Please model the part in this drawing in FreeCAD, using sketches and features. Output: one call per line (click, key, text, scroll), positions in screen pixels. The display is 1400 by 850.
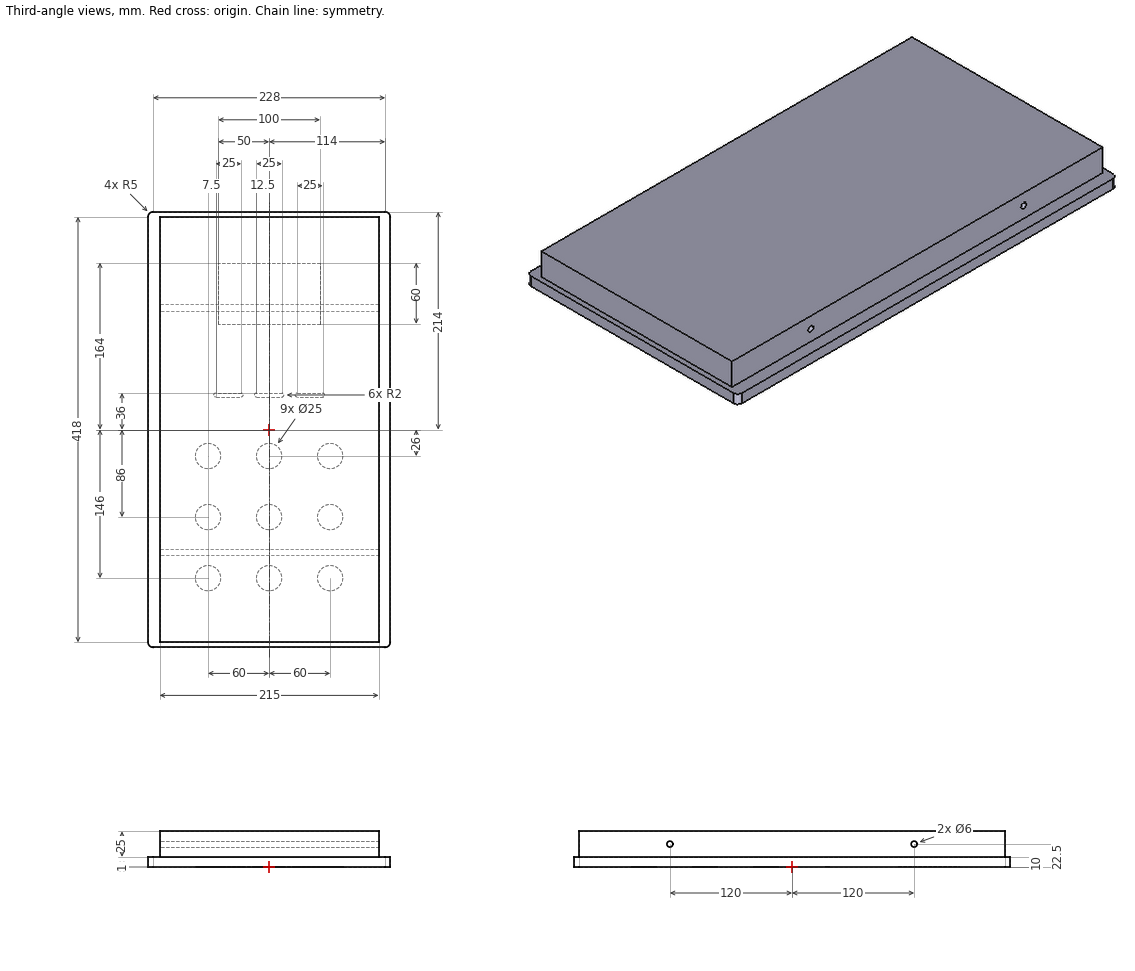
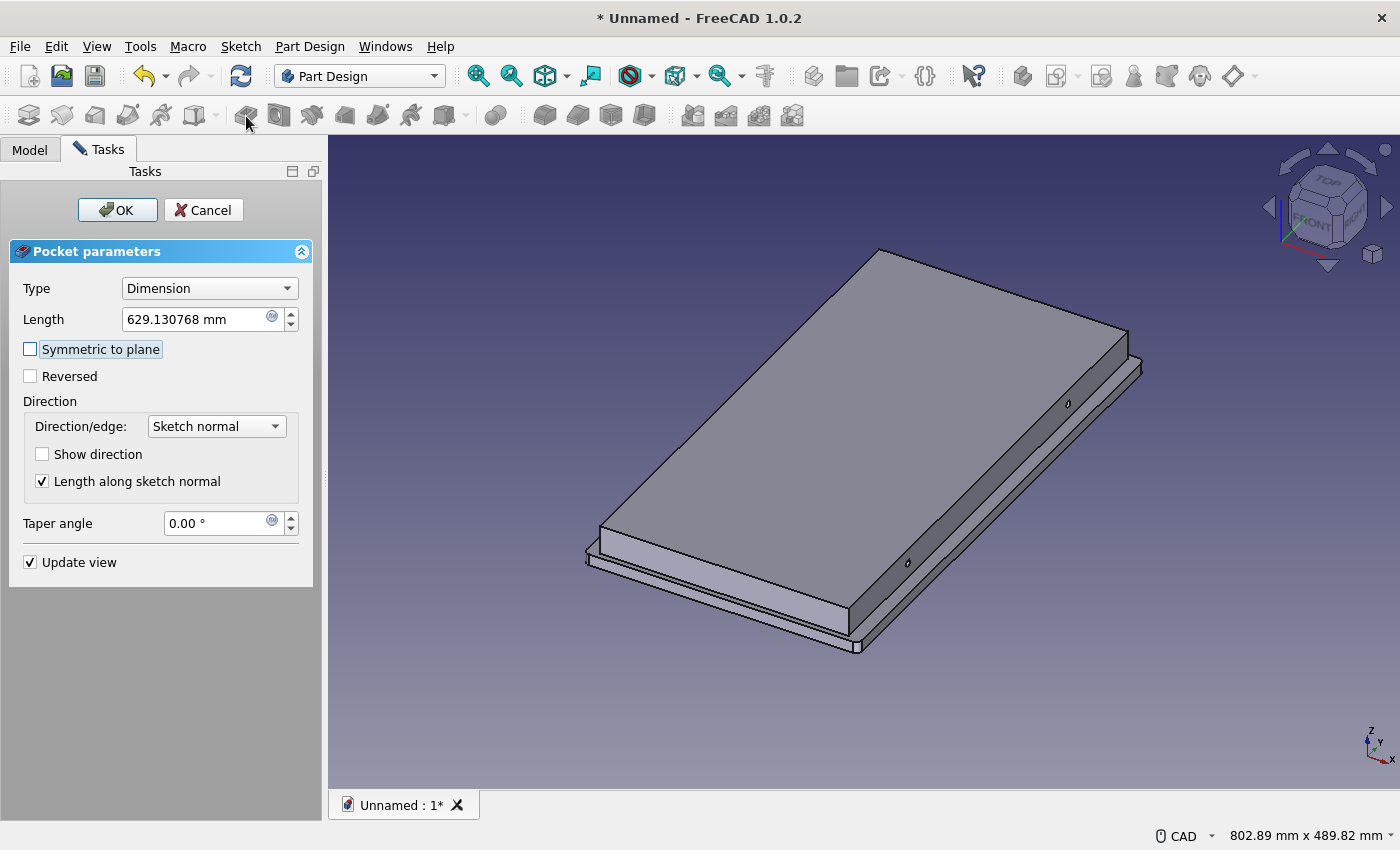
click(31, 349)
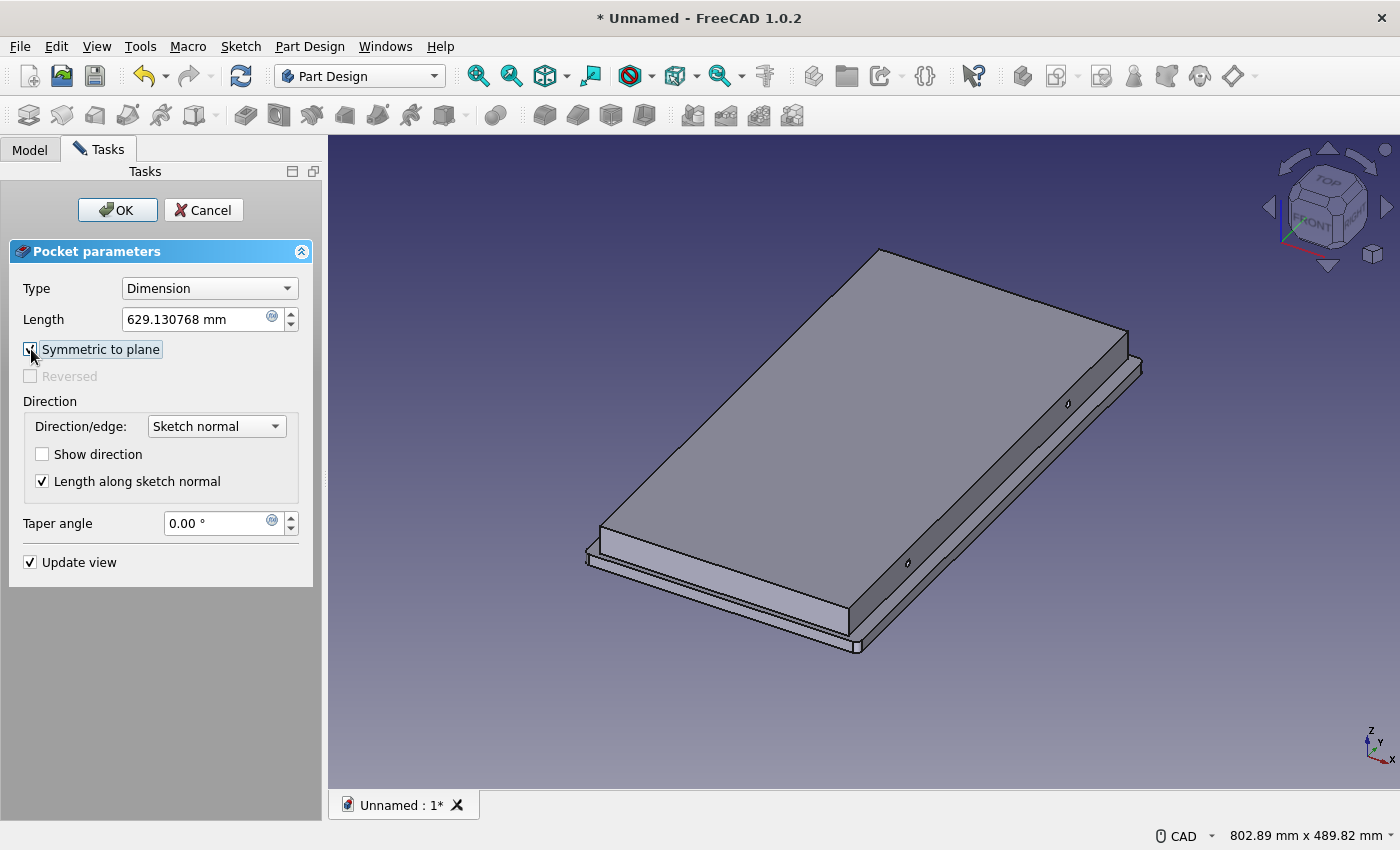
click(118, 210)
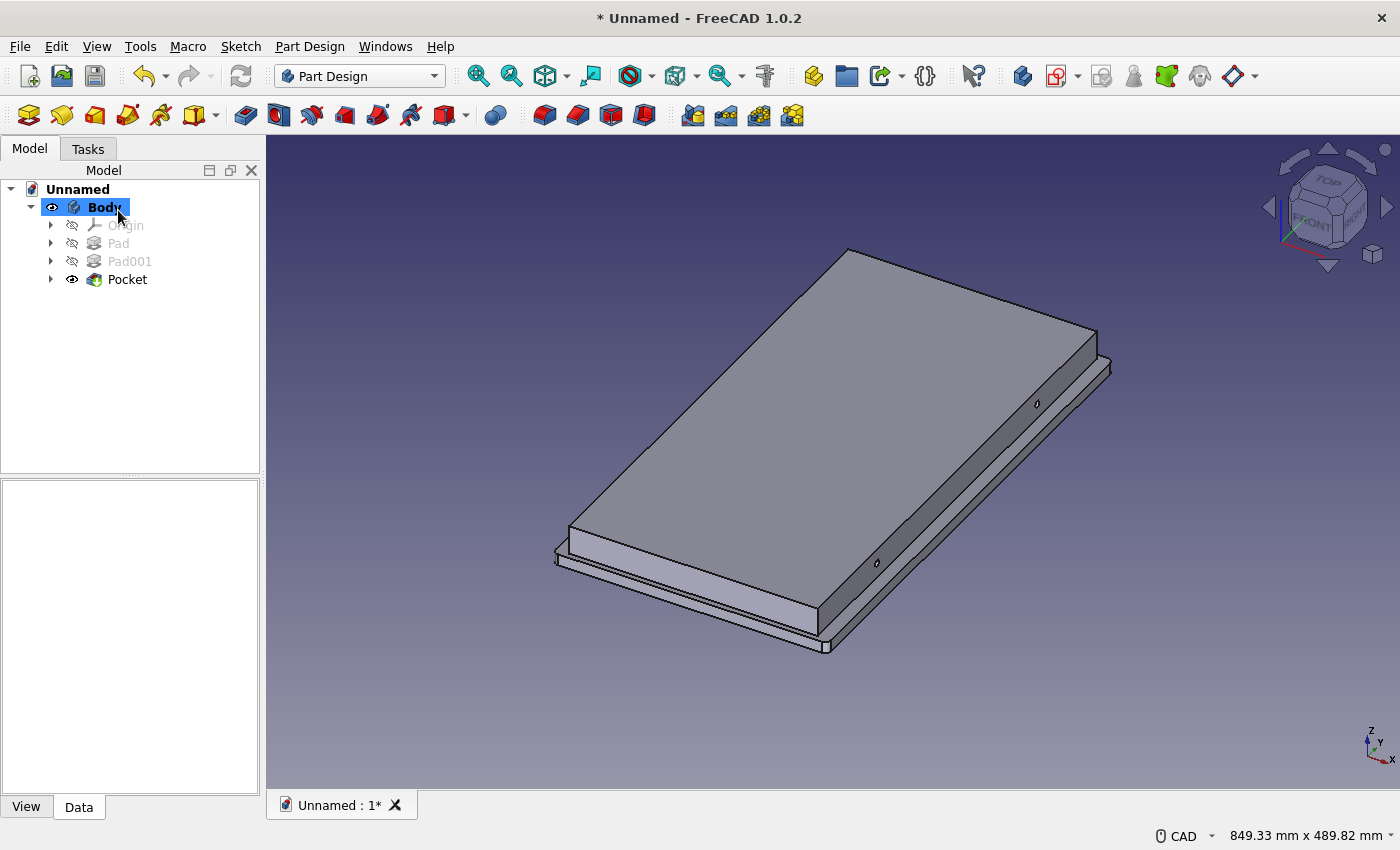
click(1056, 76)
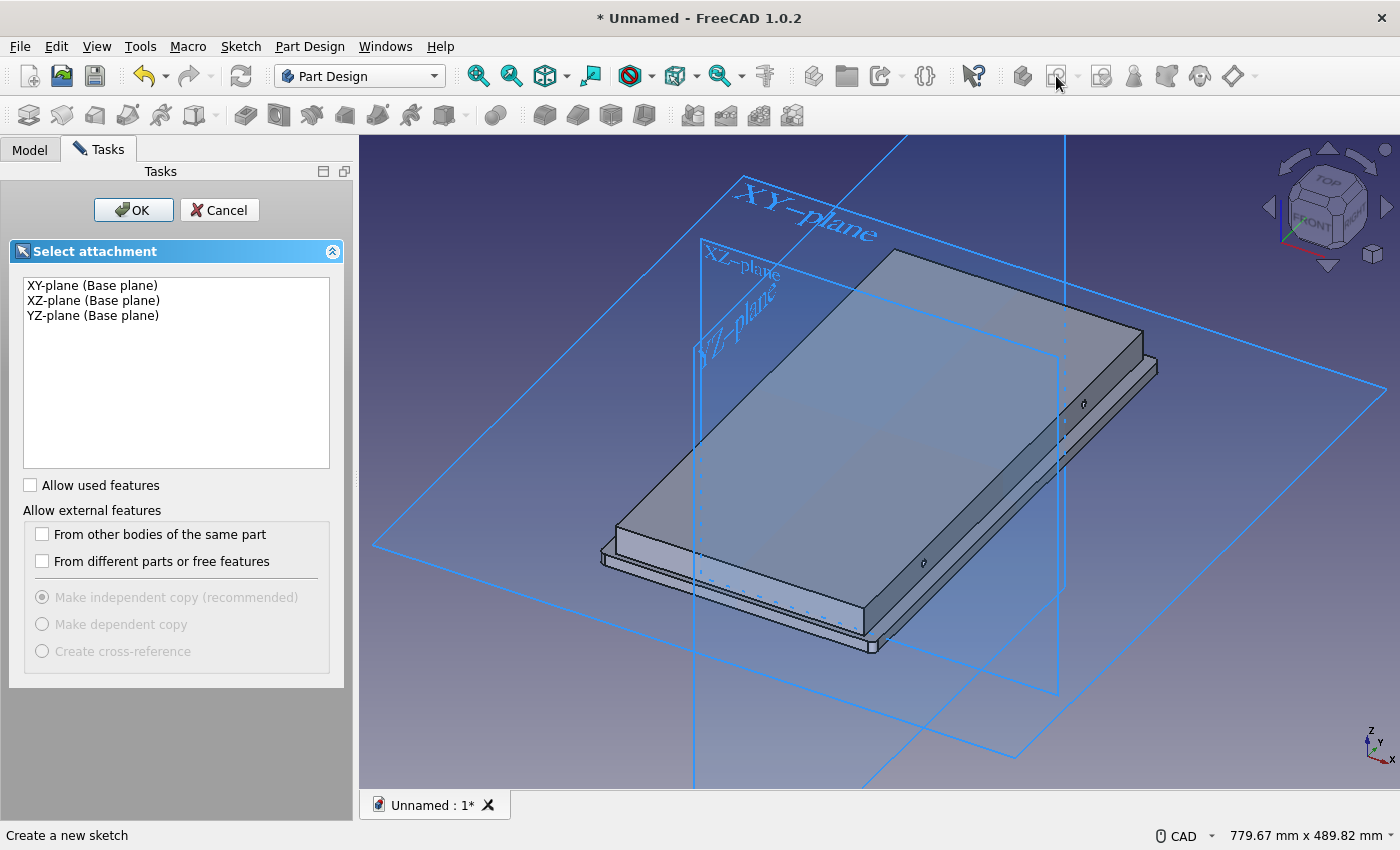
click(84, 286)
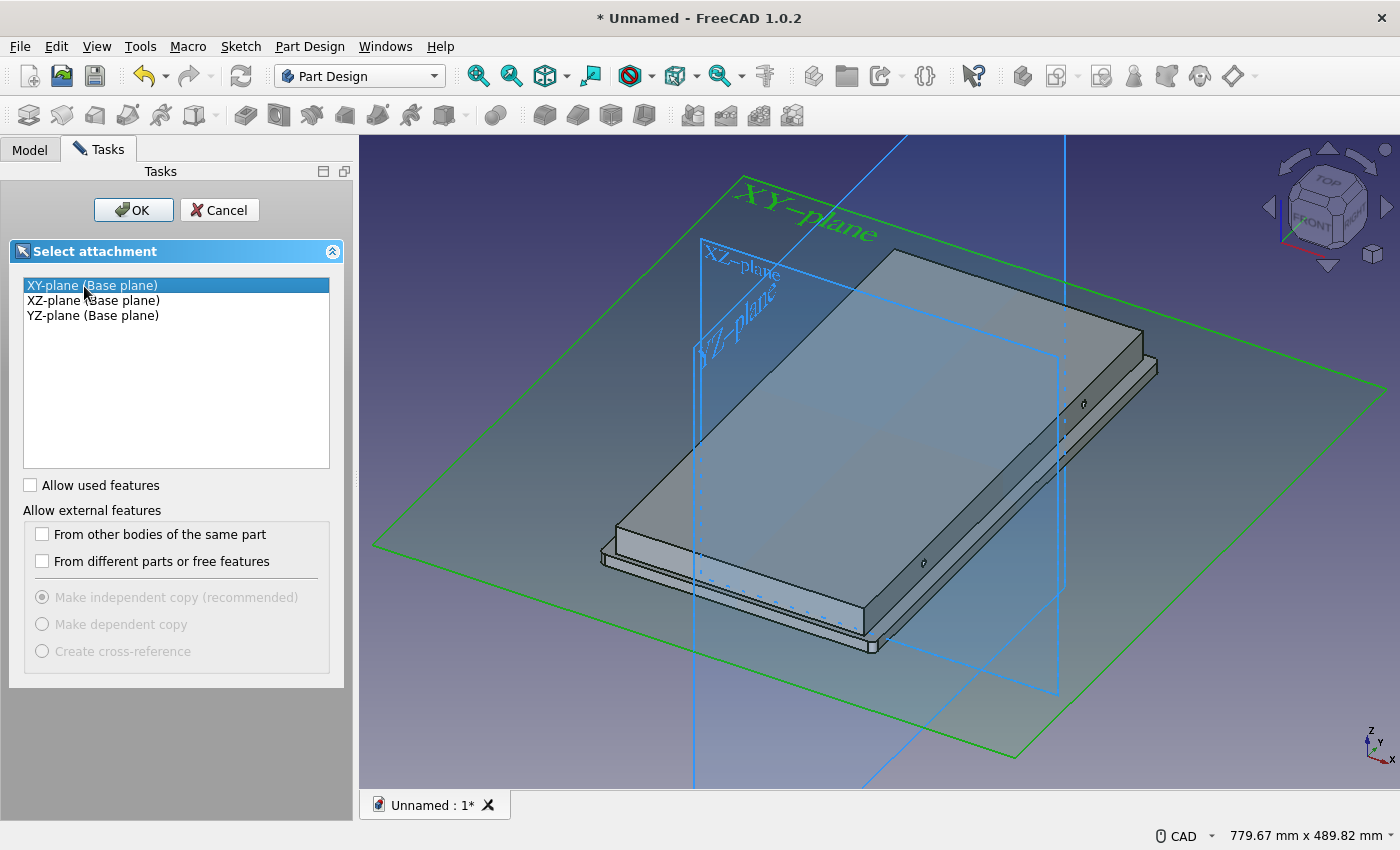
click(134, 210)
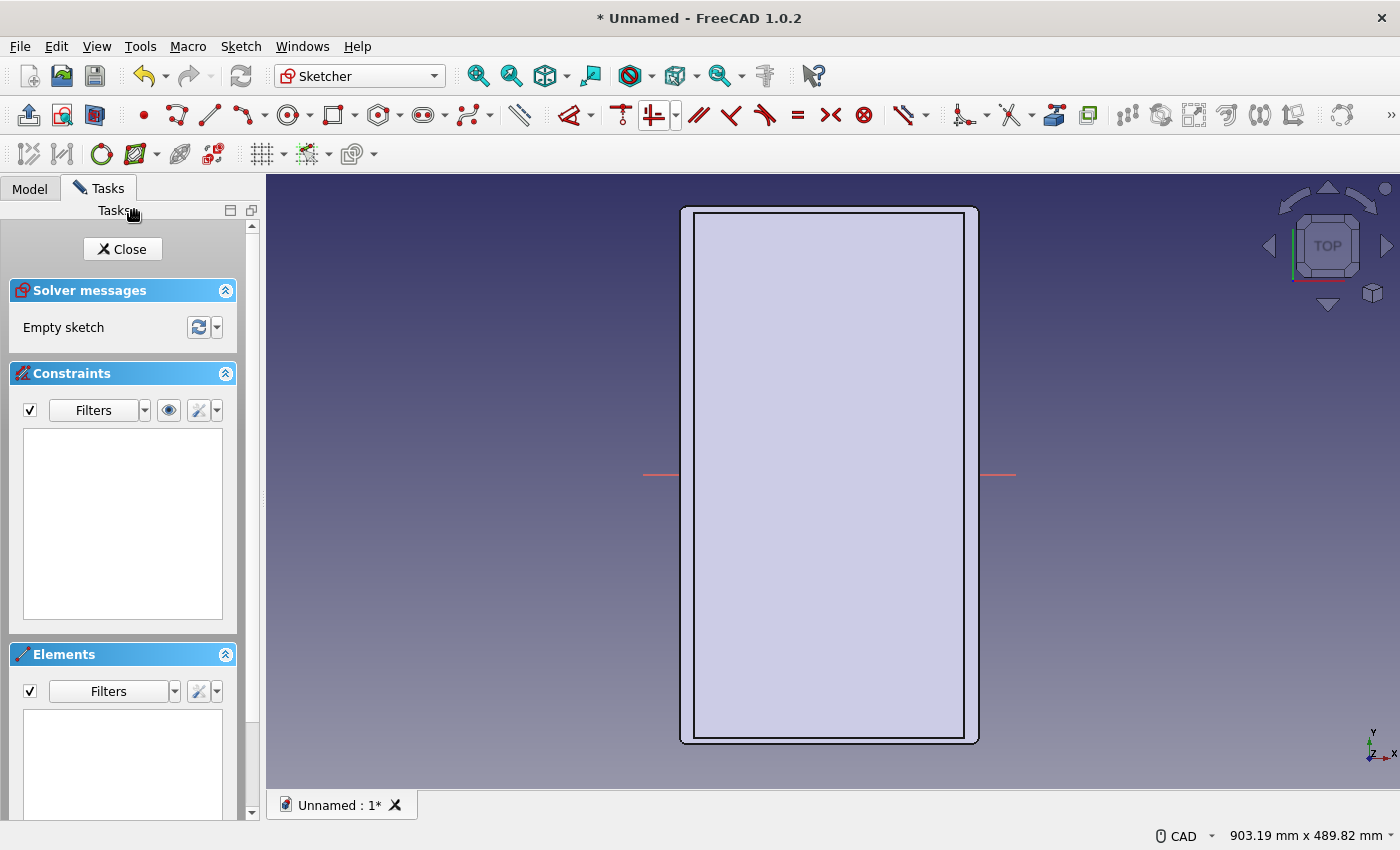
key(q)
key(s)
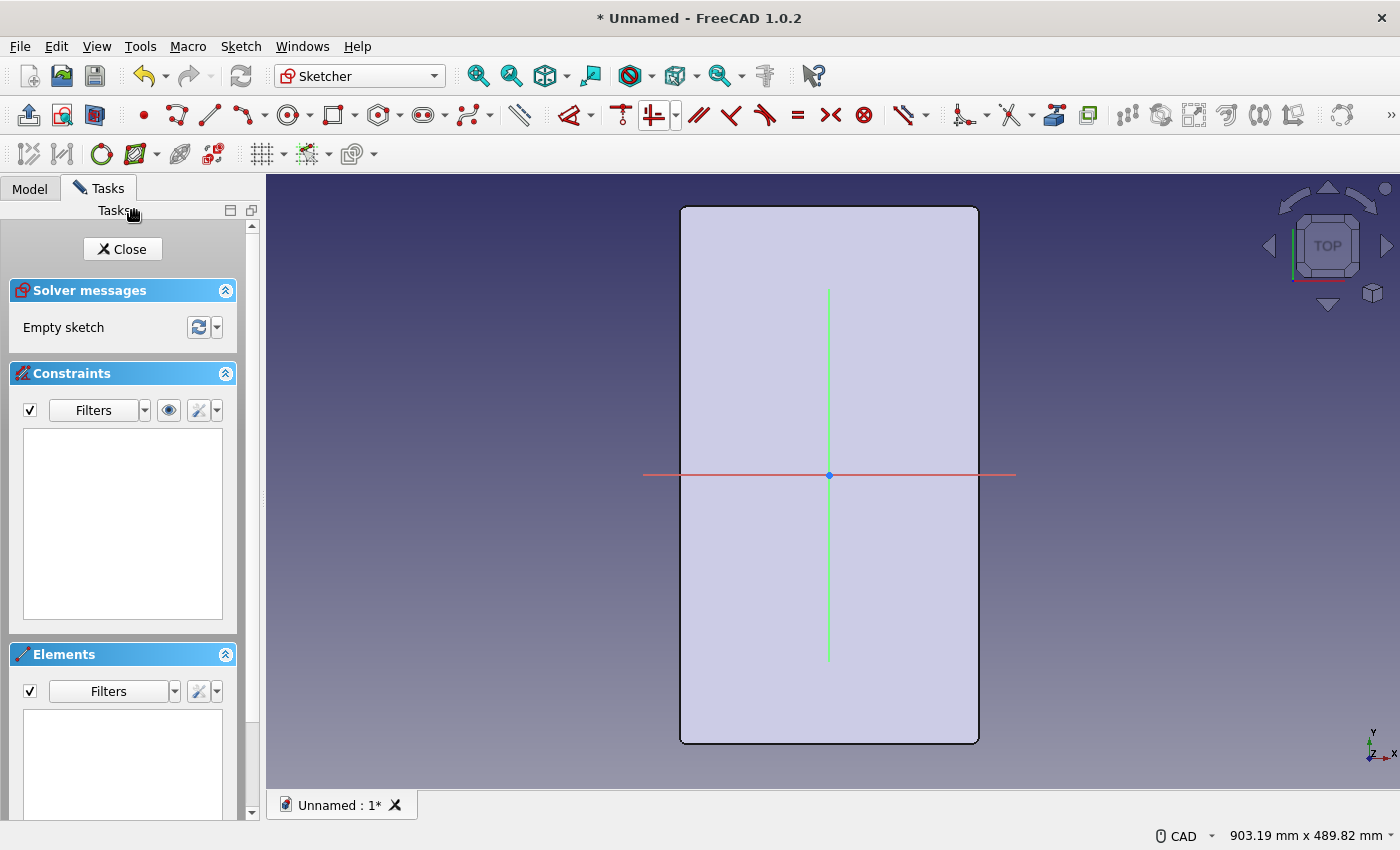
click(332, 116)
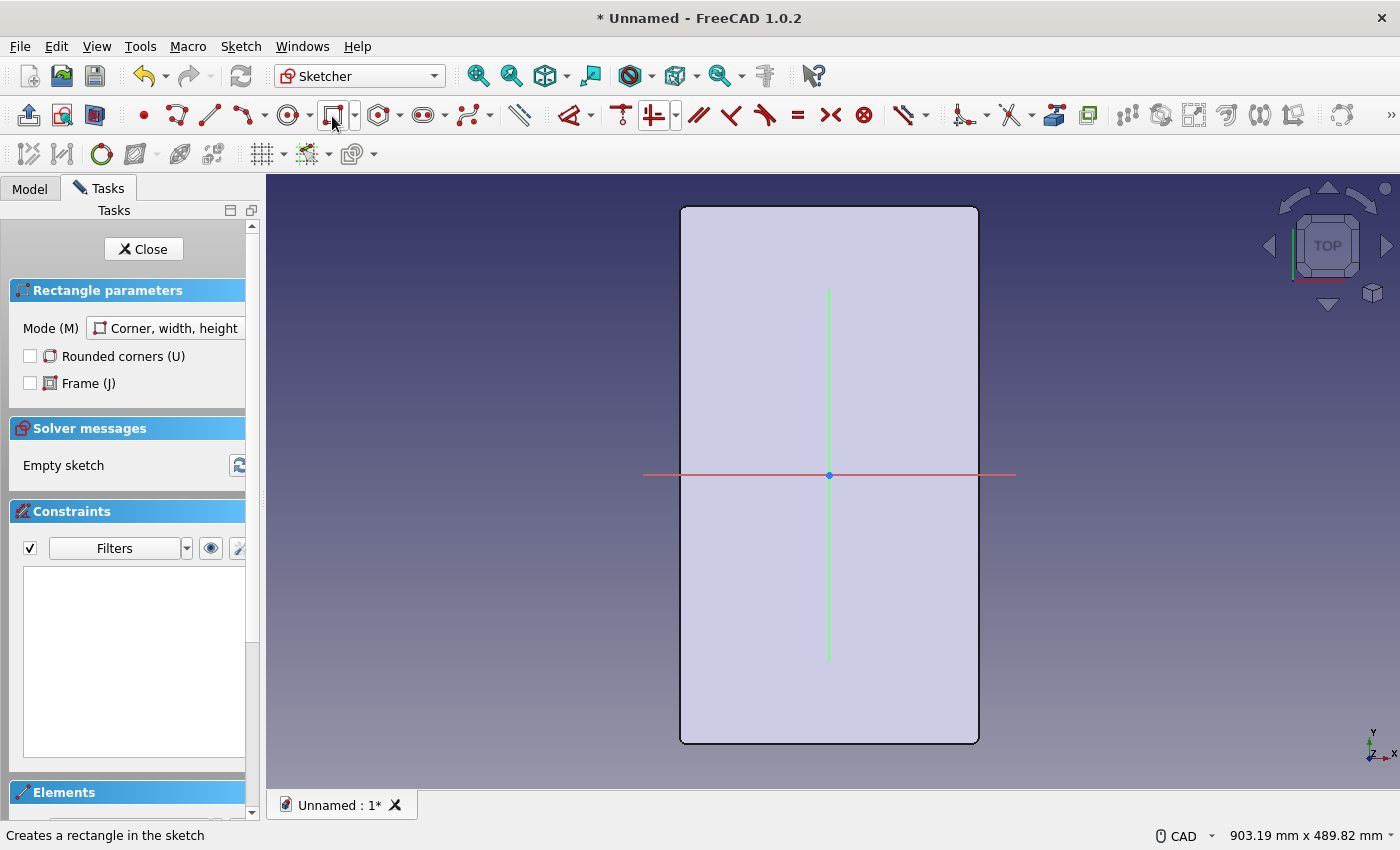
click(767, 269)
move(892, 345)